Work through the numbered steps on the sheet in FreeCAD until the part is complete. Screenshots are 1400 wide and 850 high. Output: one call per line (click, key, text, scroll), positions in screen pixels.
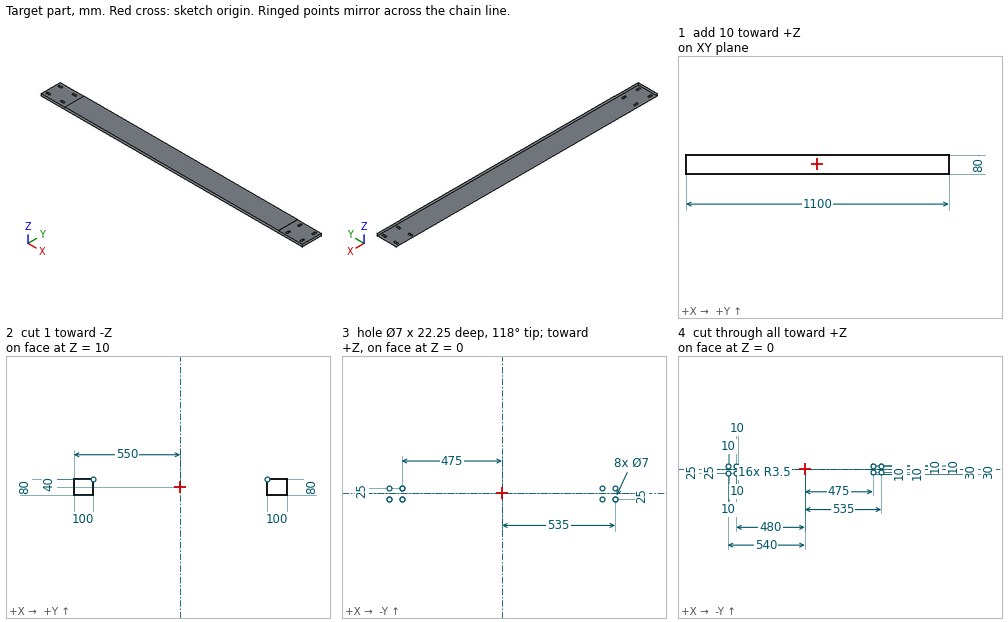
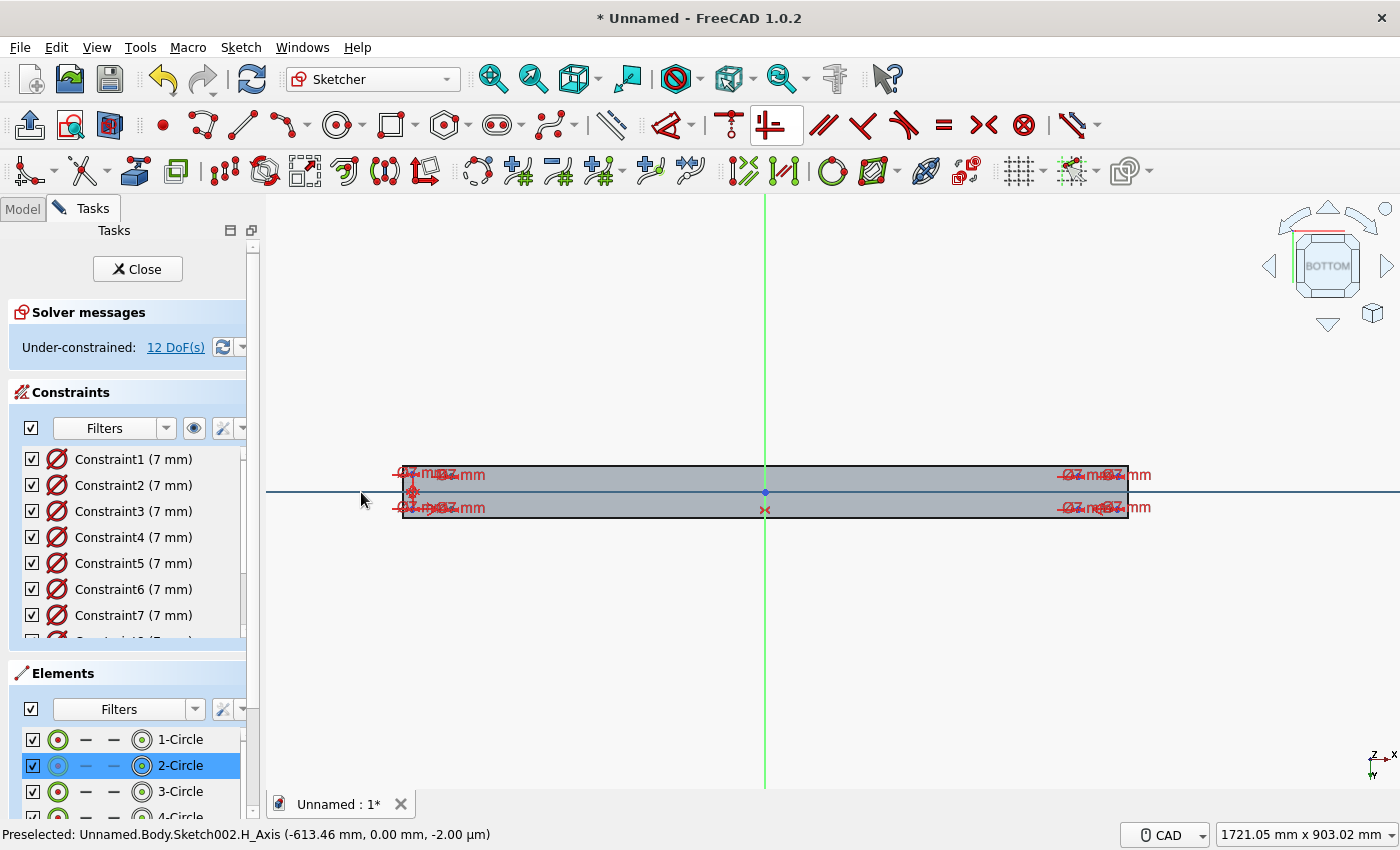
click(984, 126)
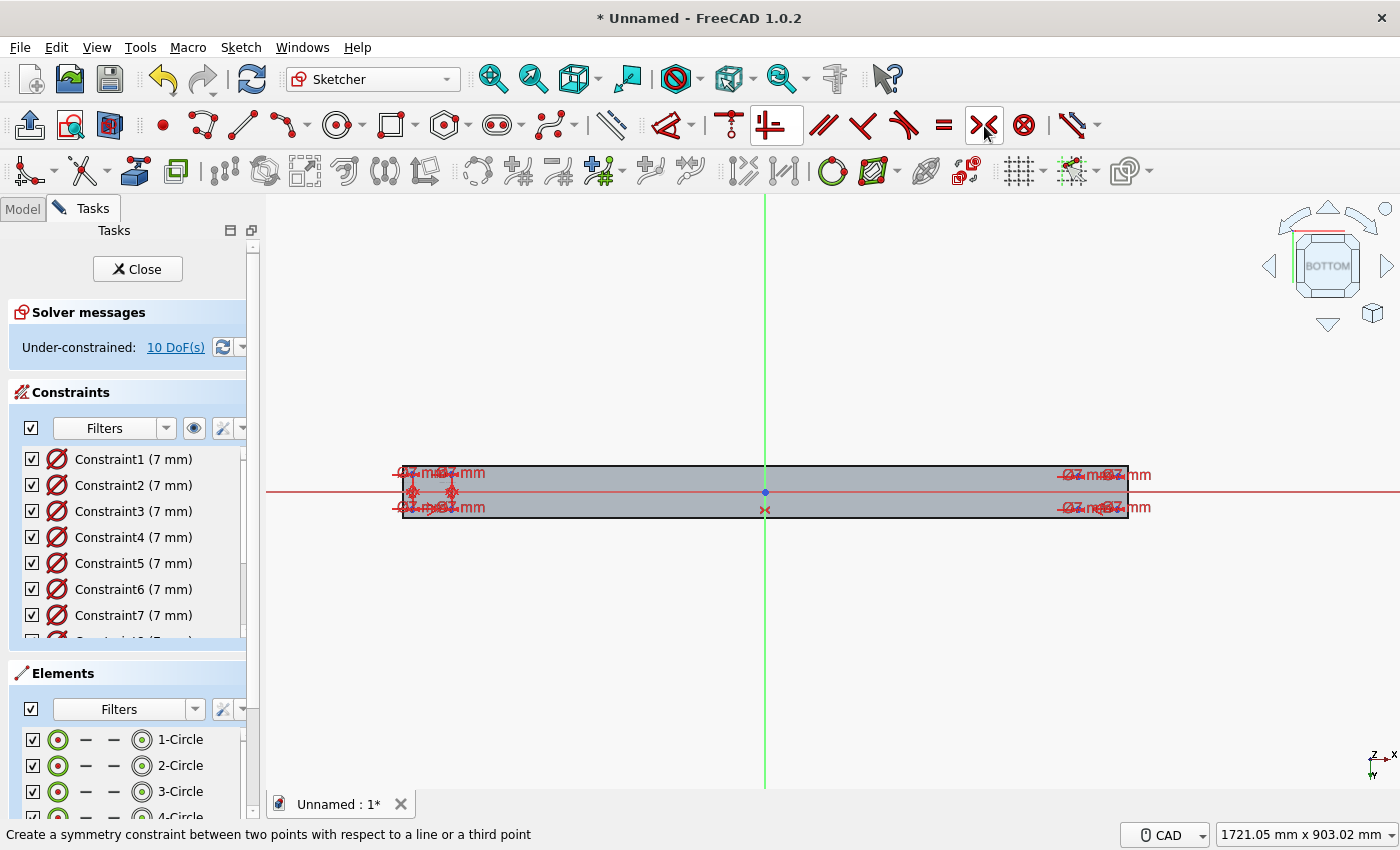
click(452, 509)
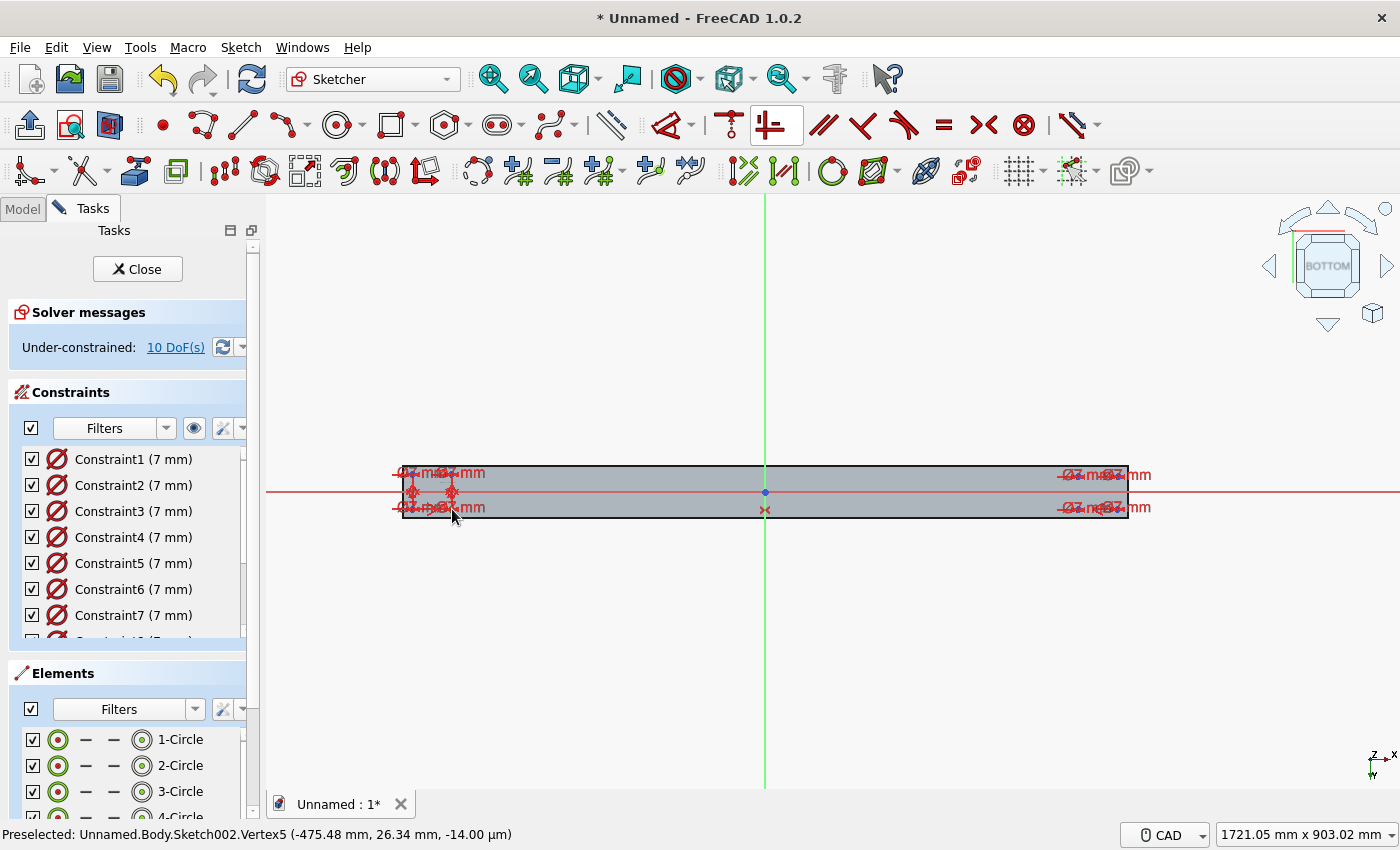
click(1078, 510)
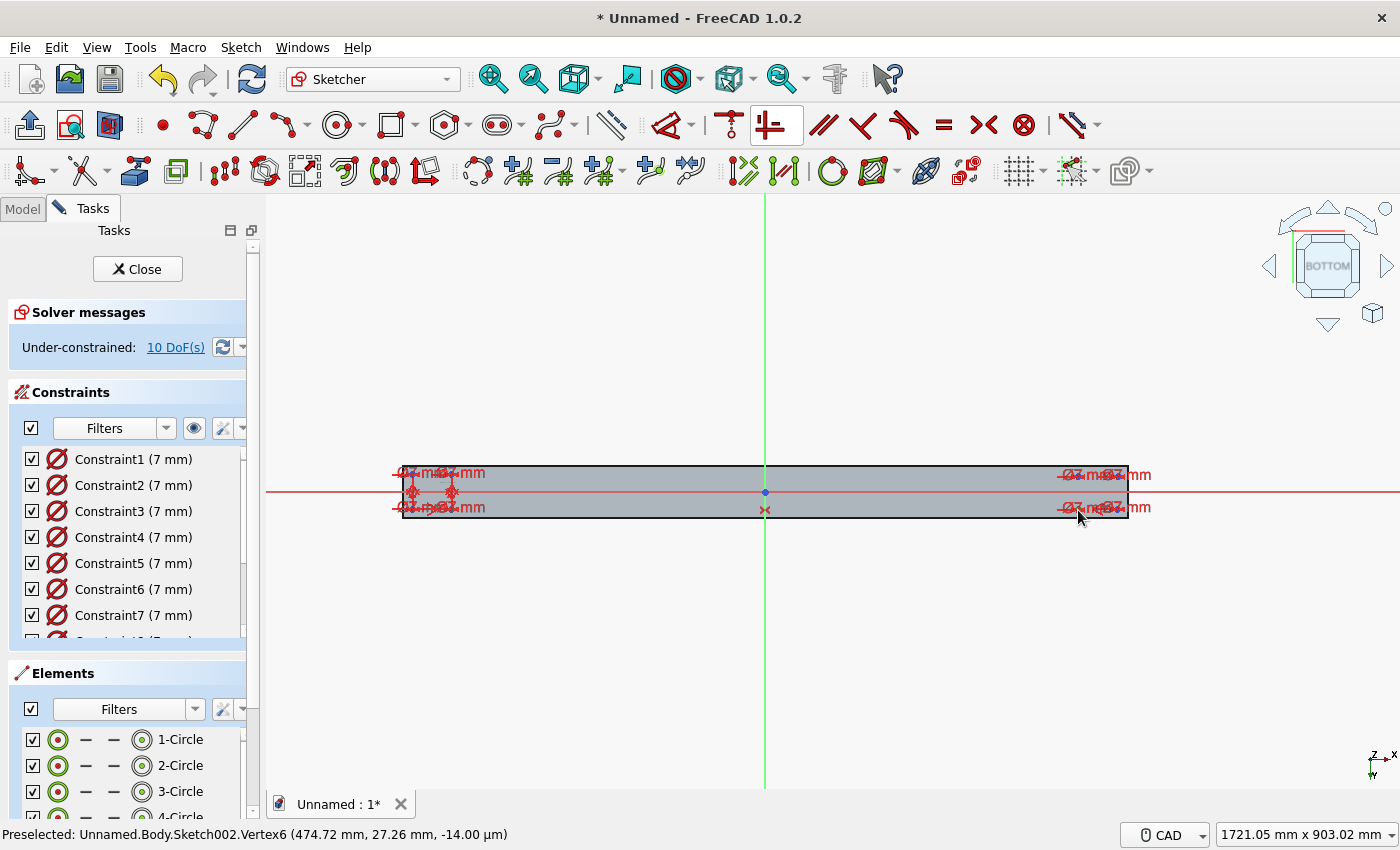
click(765, 722)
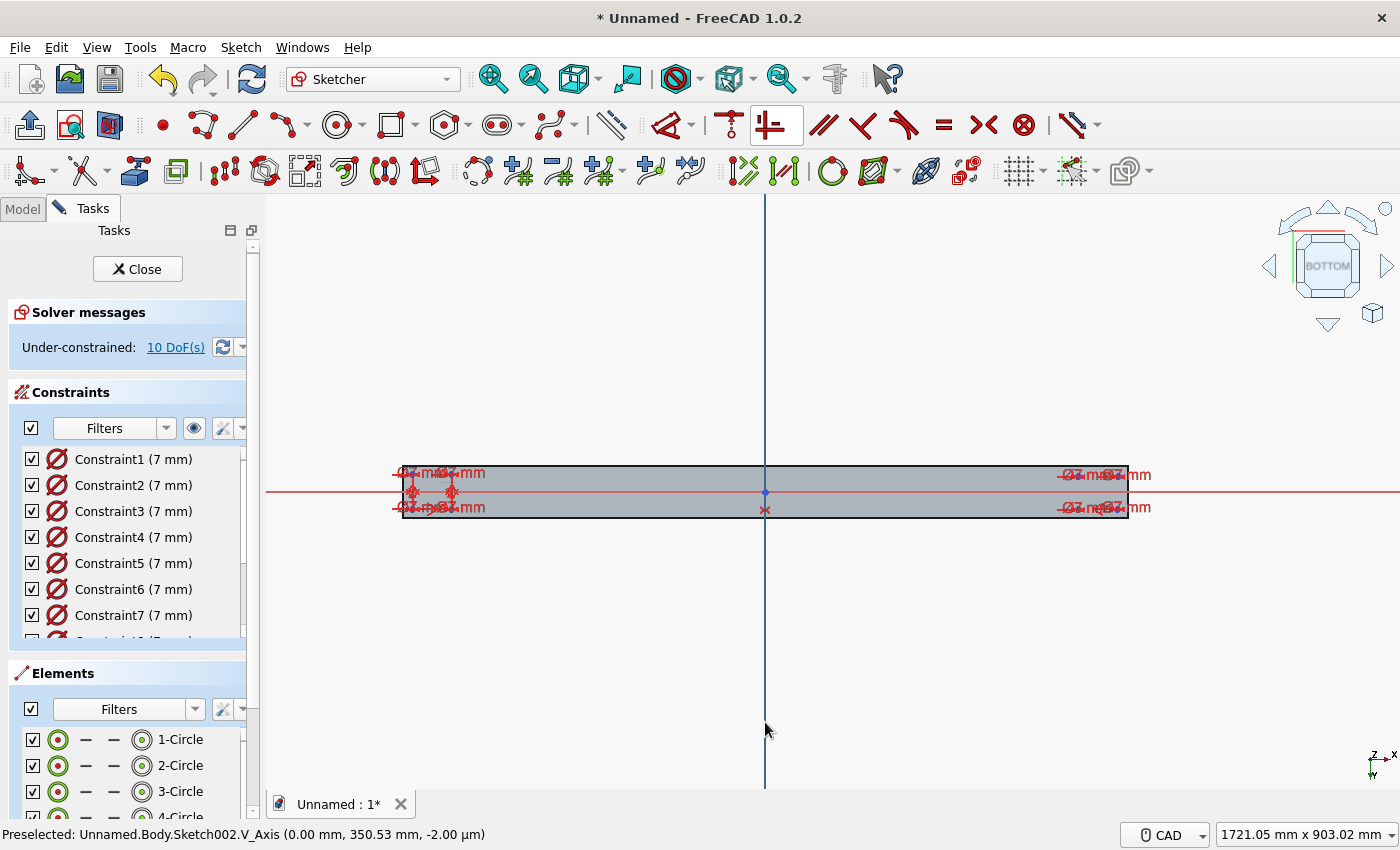
click(984, 126)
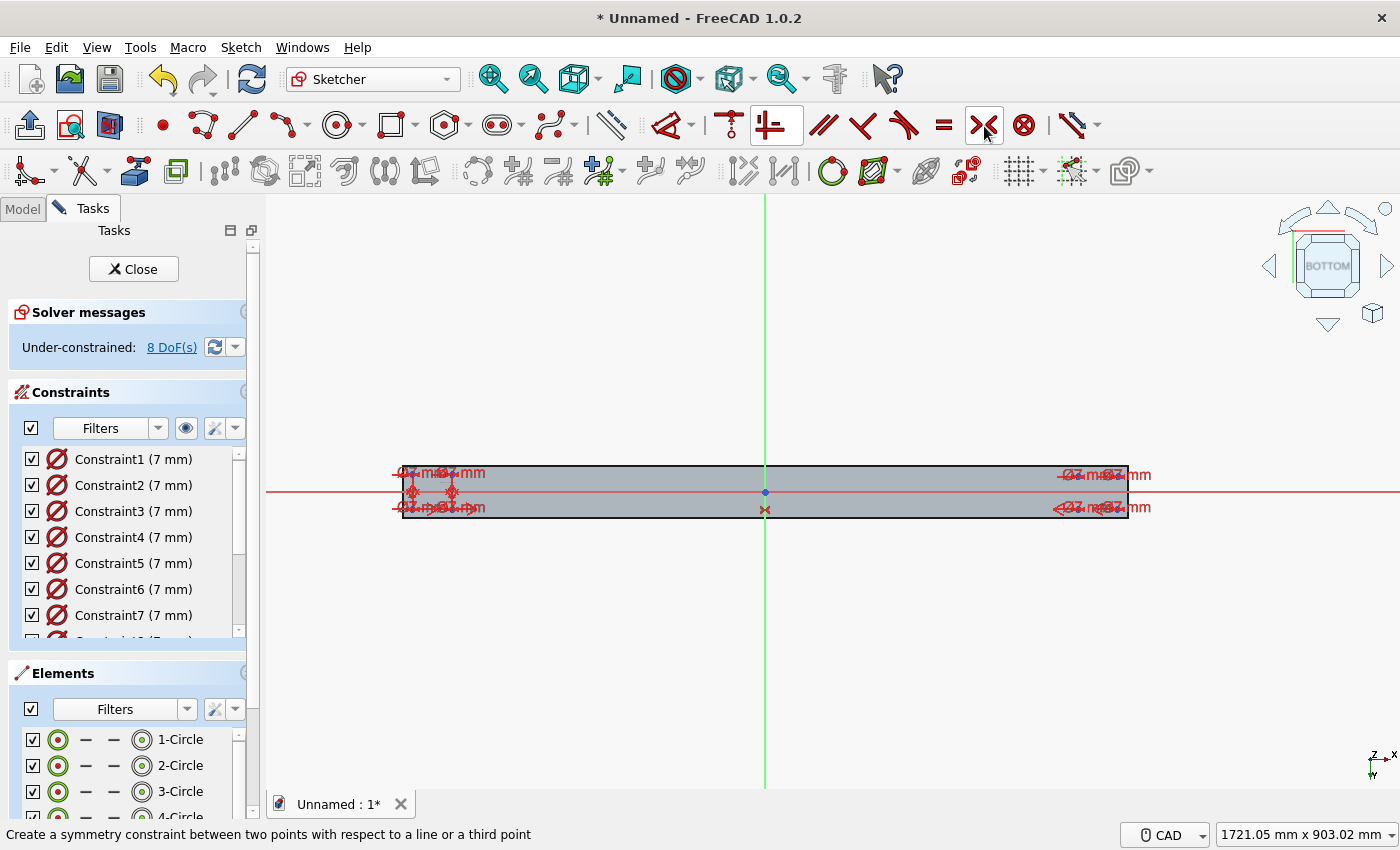
click(452, 475)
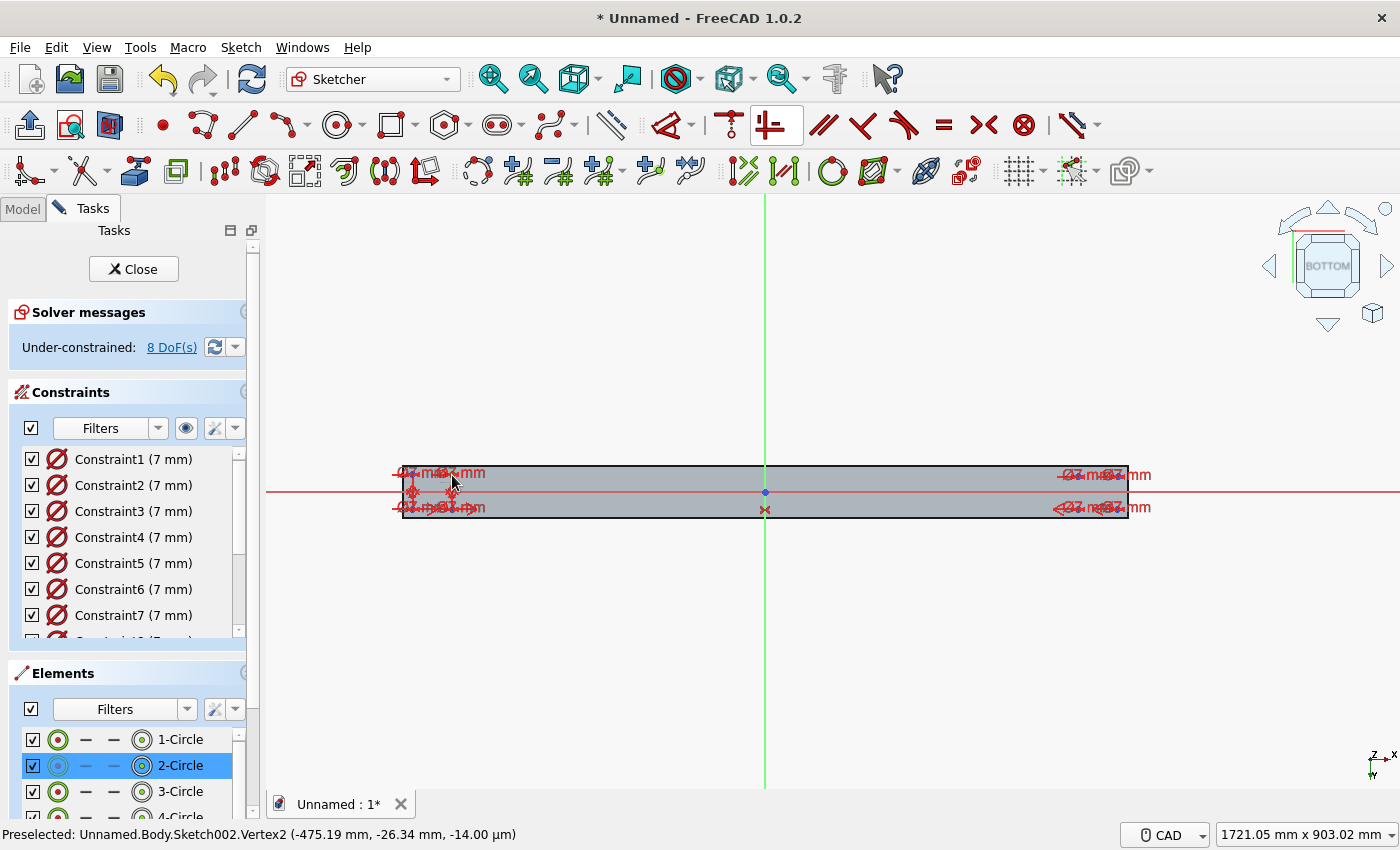
click(1078, 477)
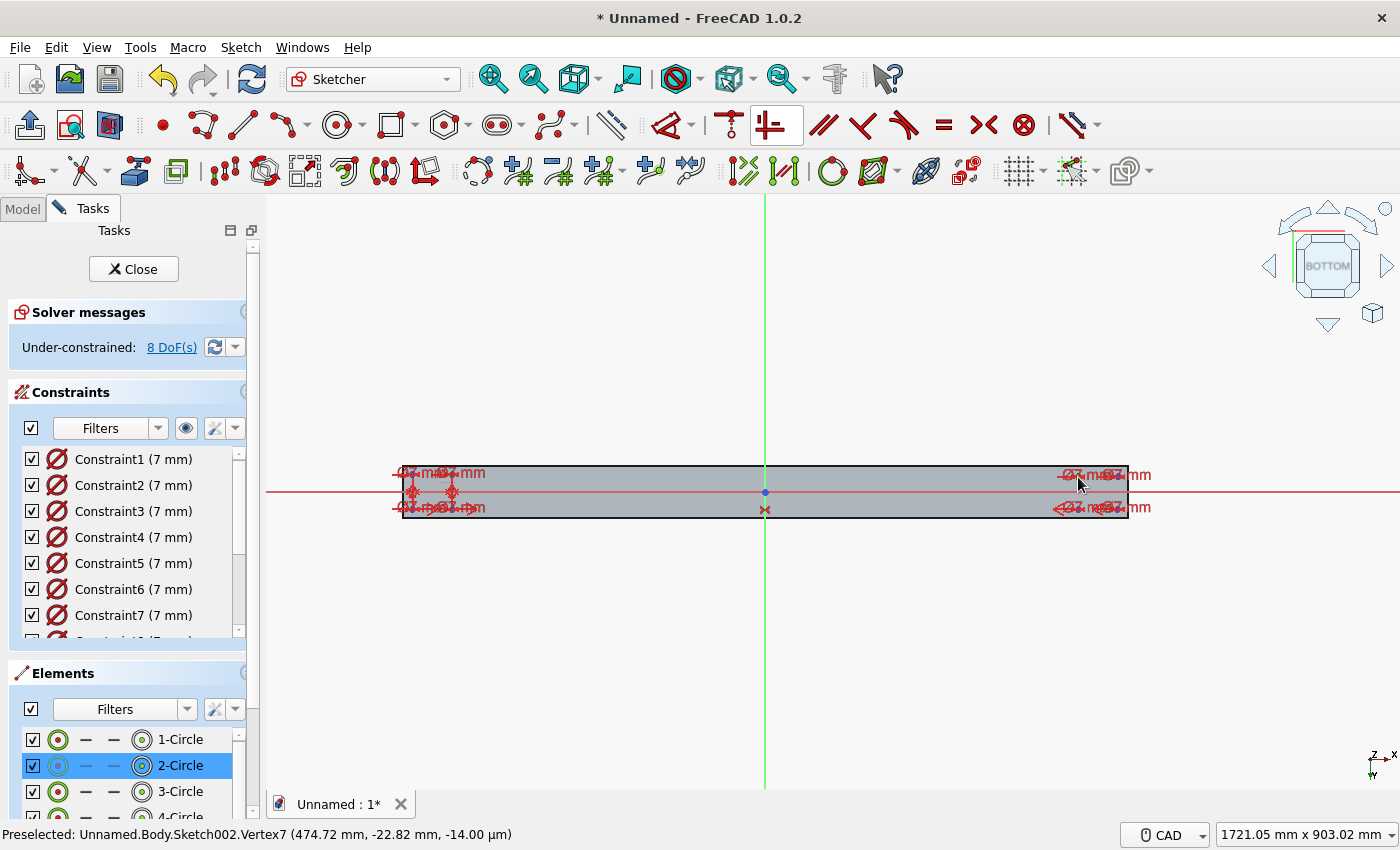
click(765, 722)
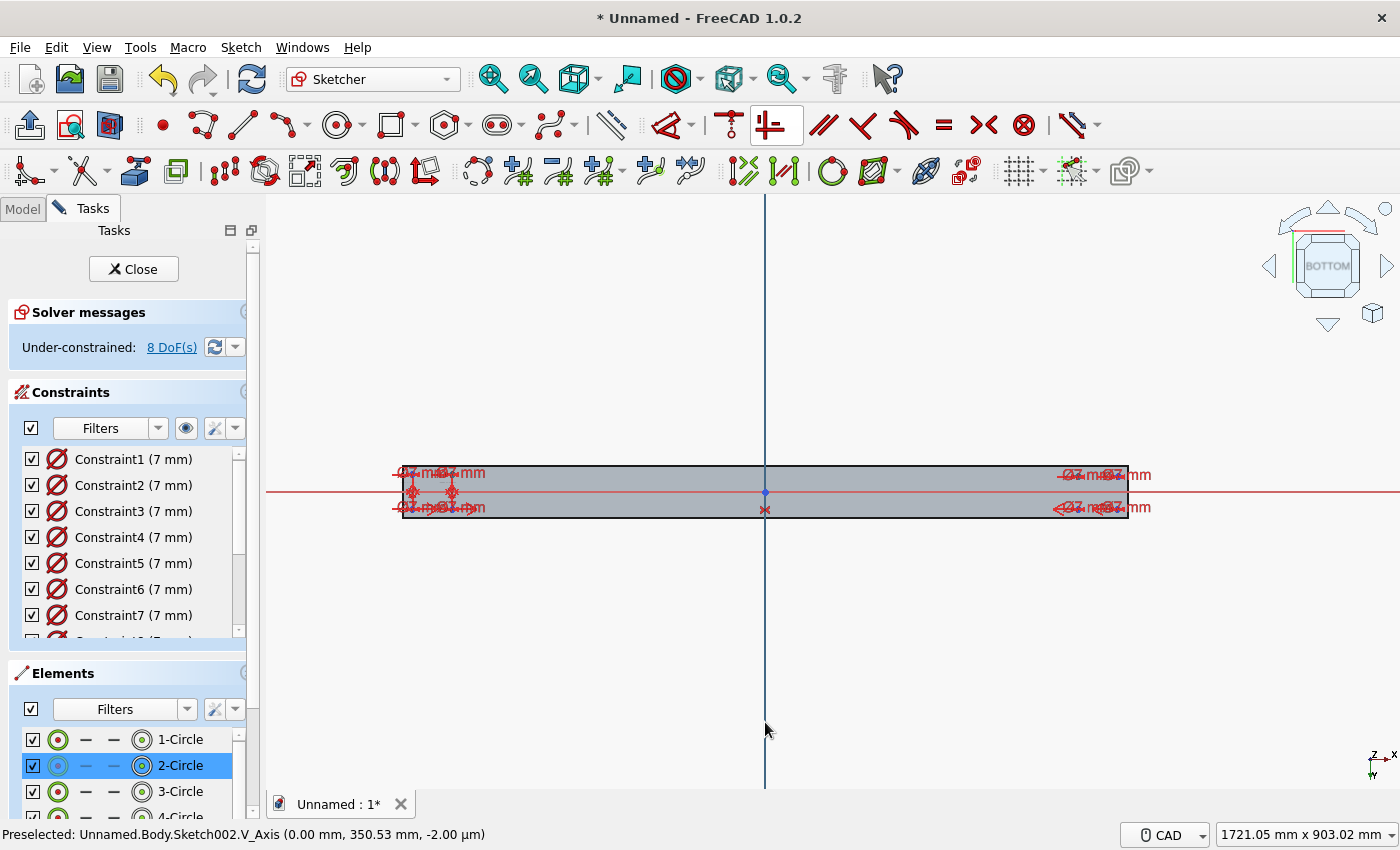
click(984, 126)